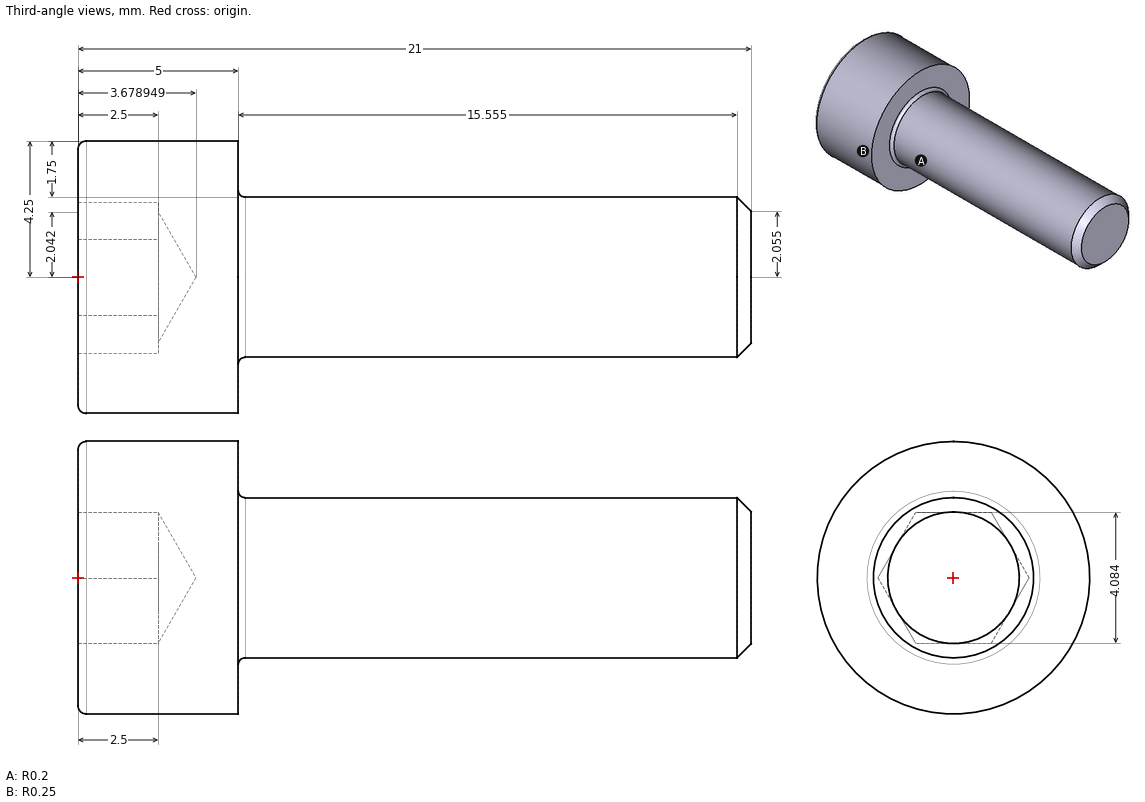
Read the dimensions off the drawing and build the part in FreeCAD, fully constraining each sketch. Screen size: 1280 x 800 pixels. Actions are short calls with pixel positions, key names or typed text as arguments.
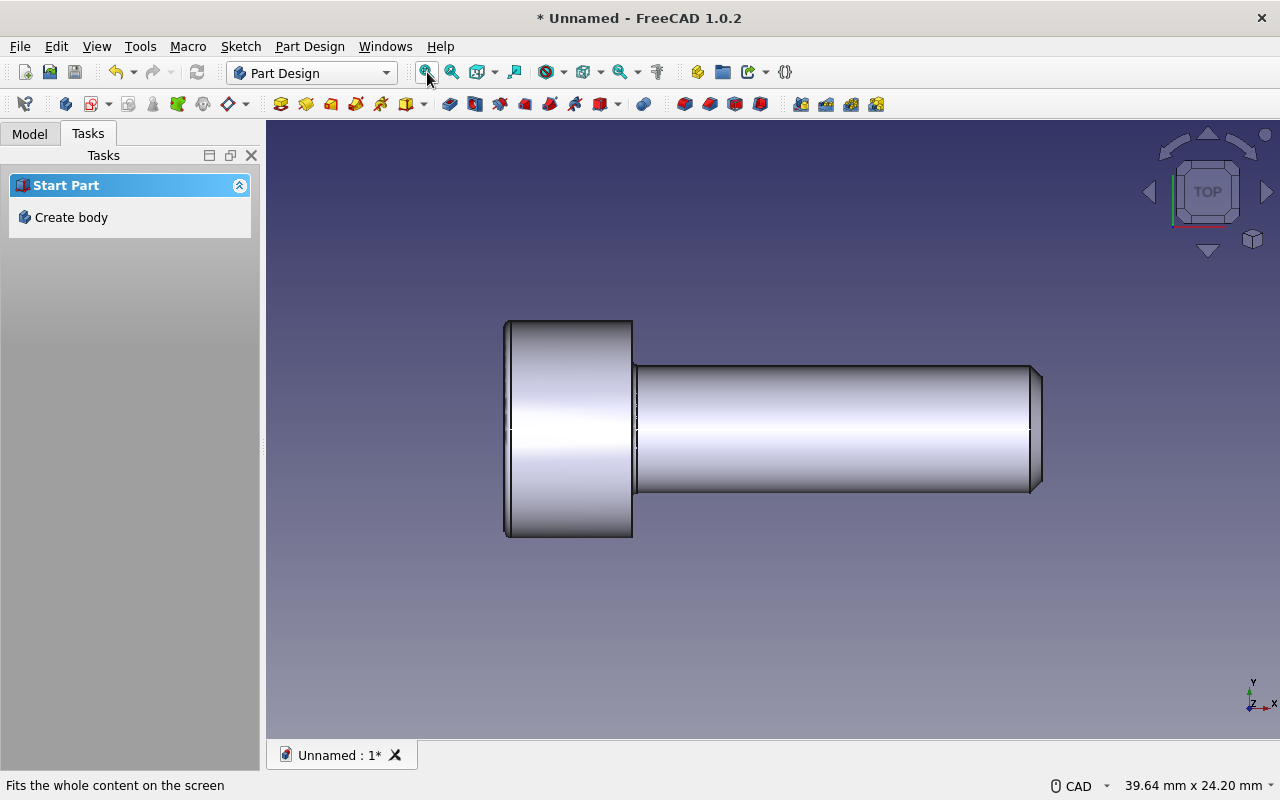
key(6)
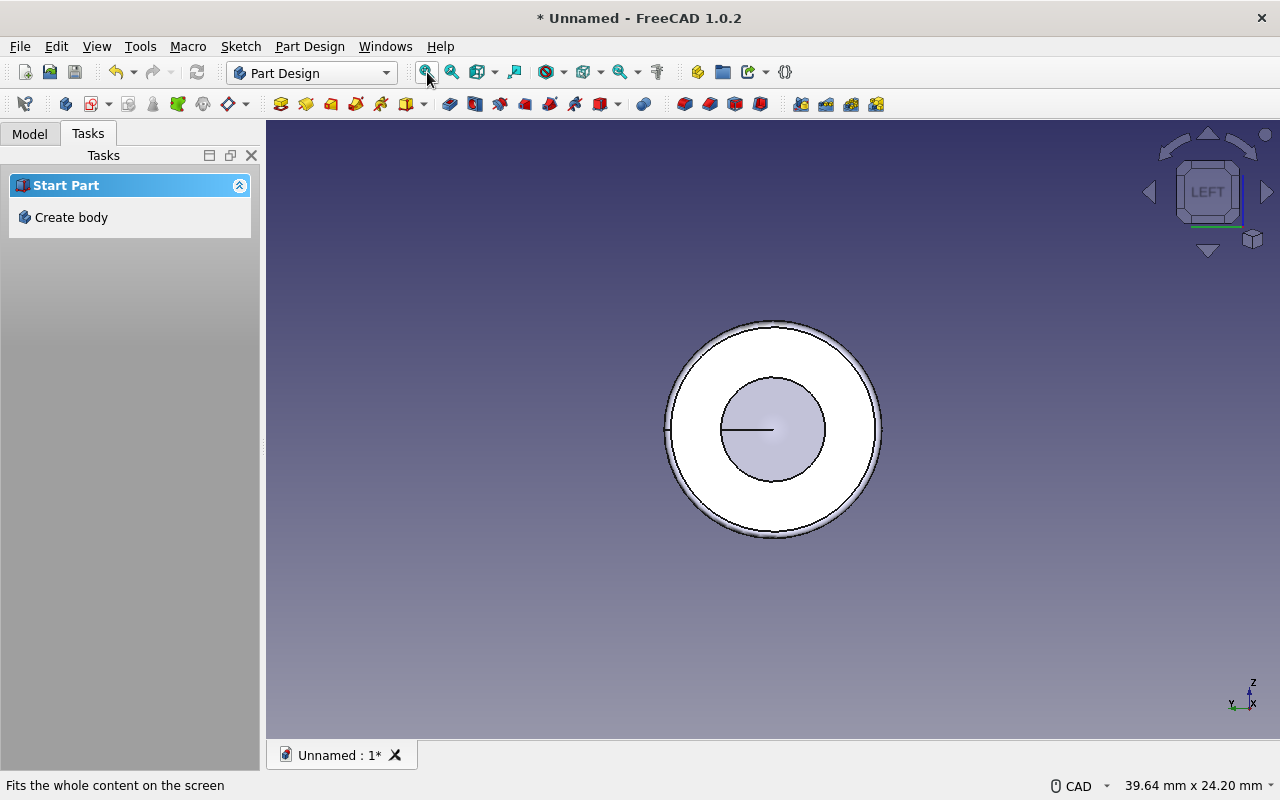
click(427, 72)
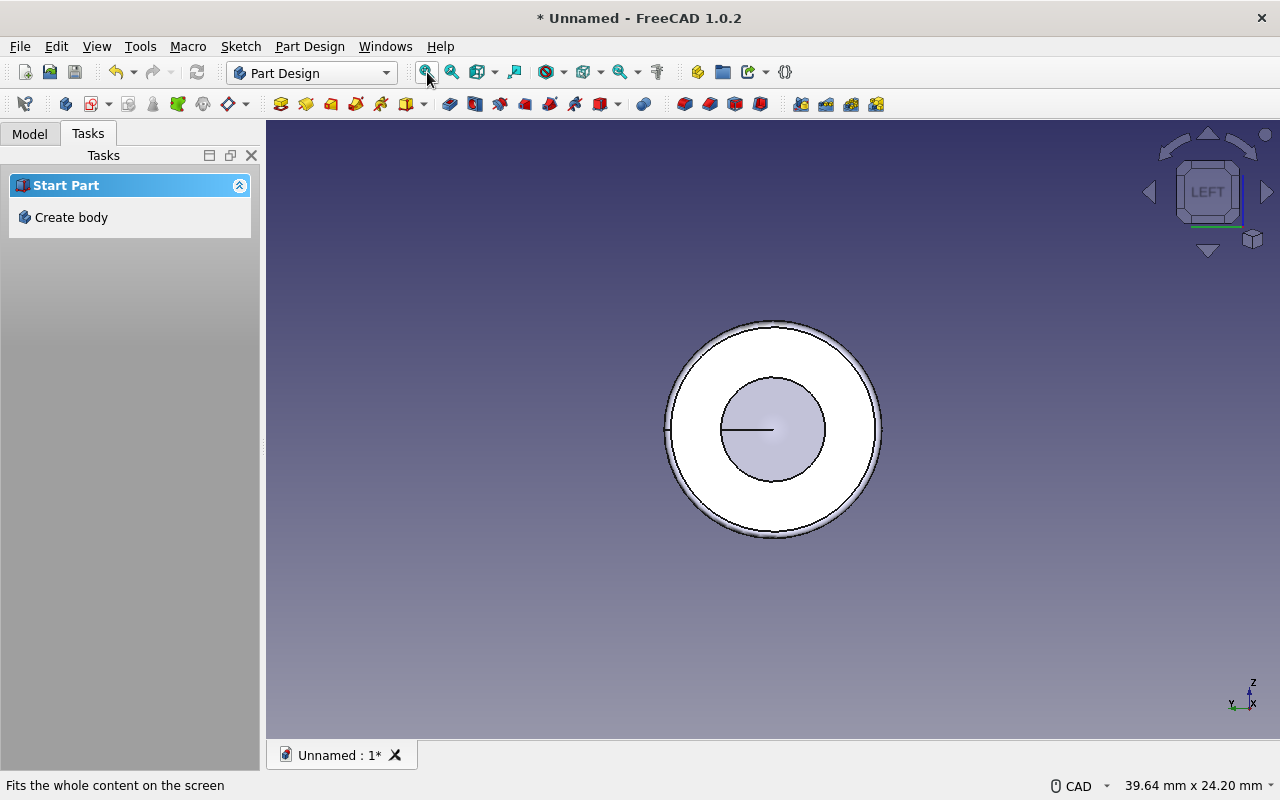
click(831, 487)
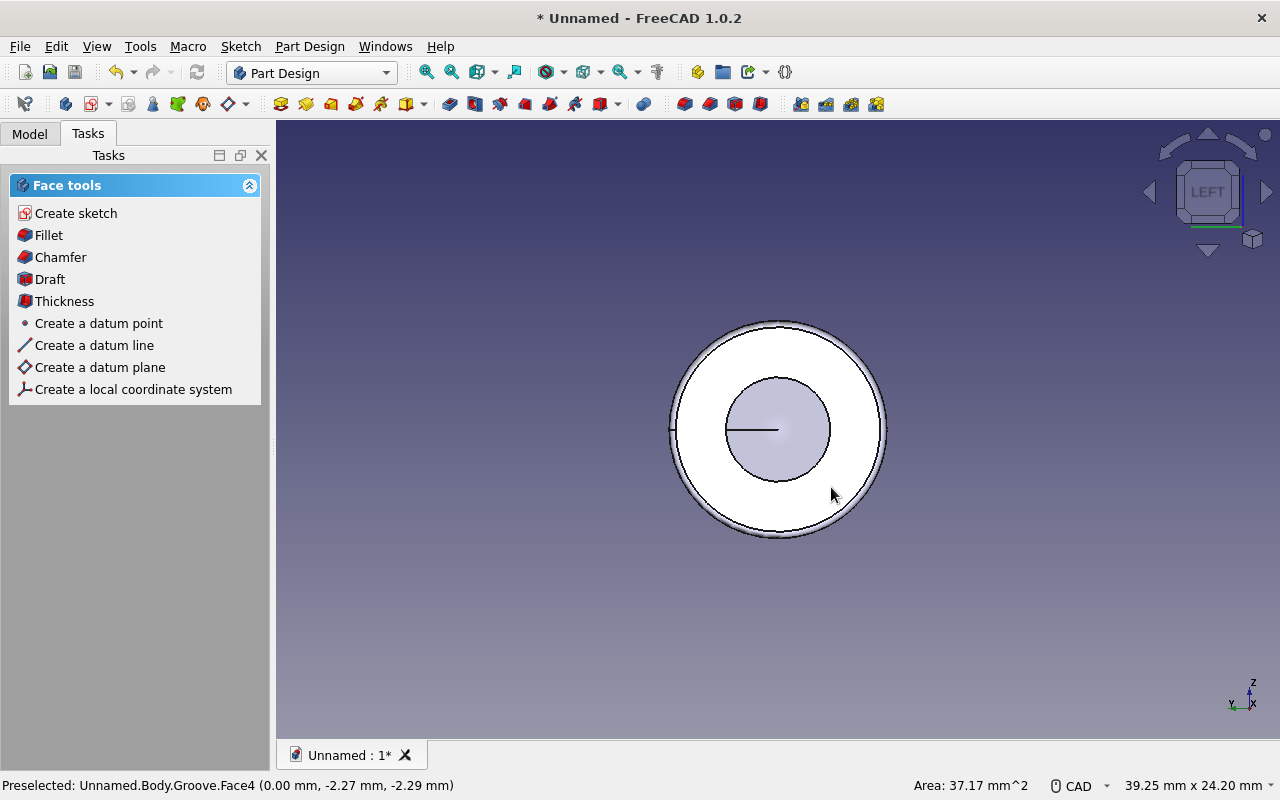
click(90, 104)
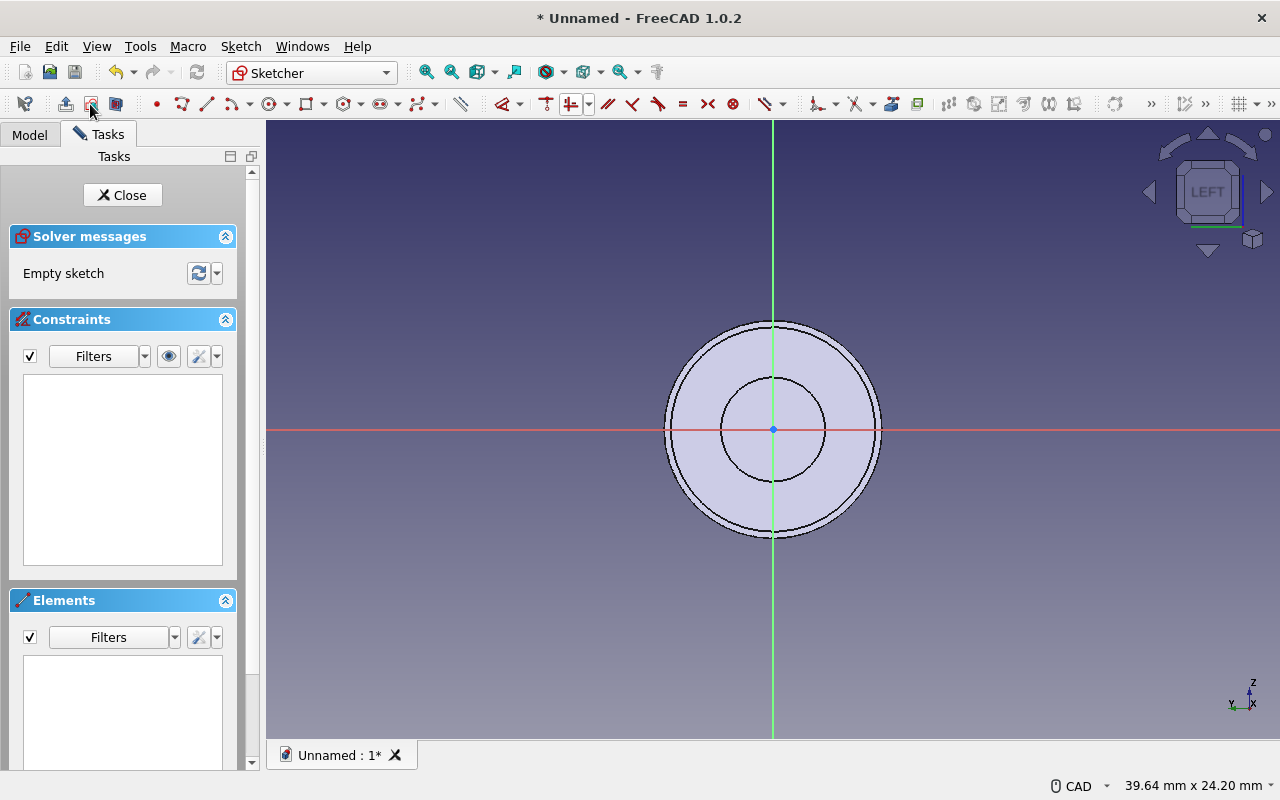
scroll(795, 430, up, 7)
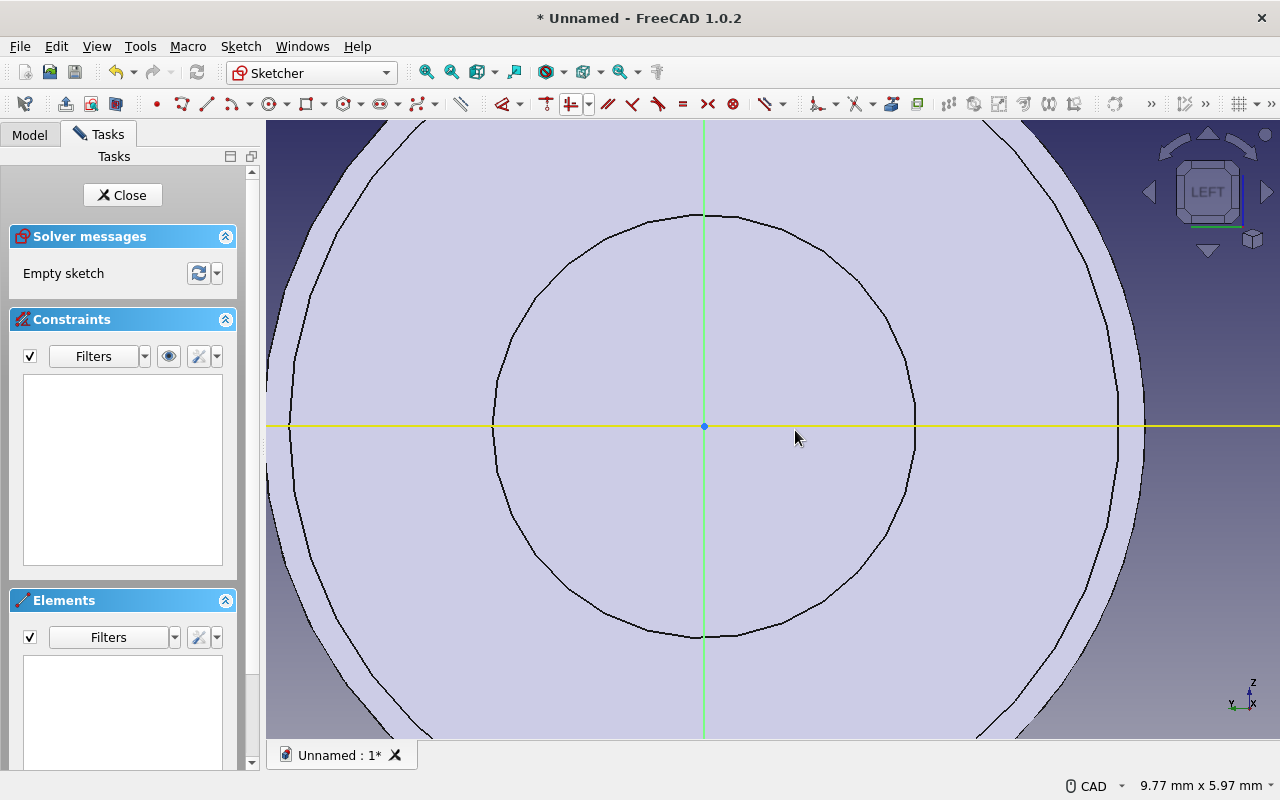
click(342, 104)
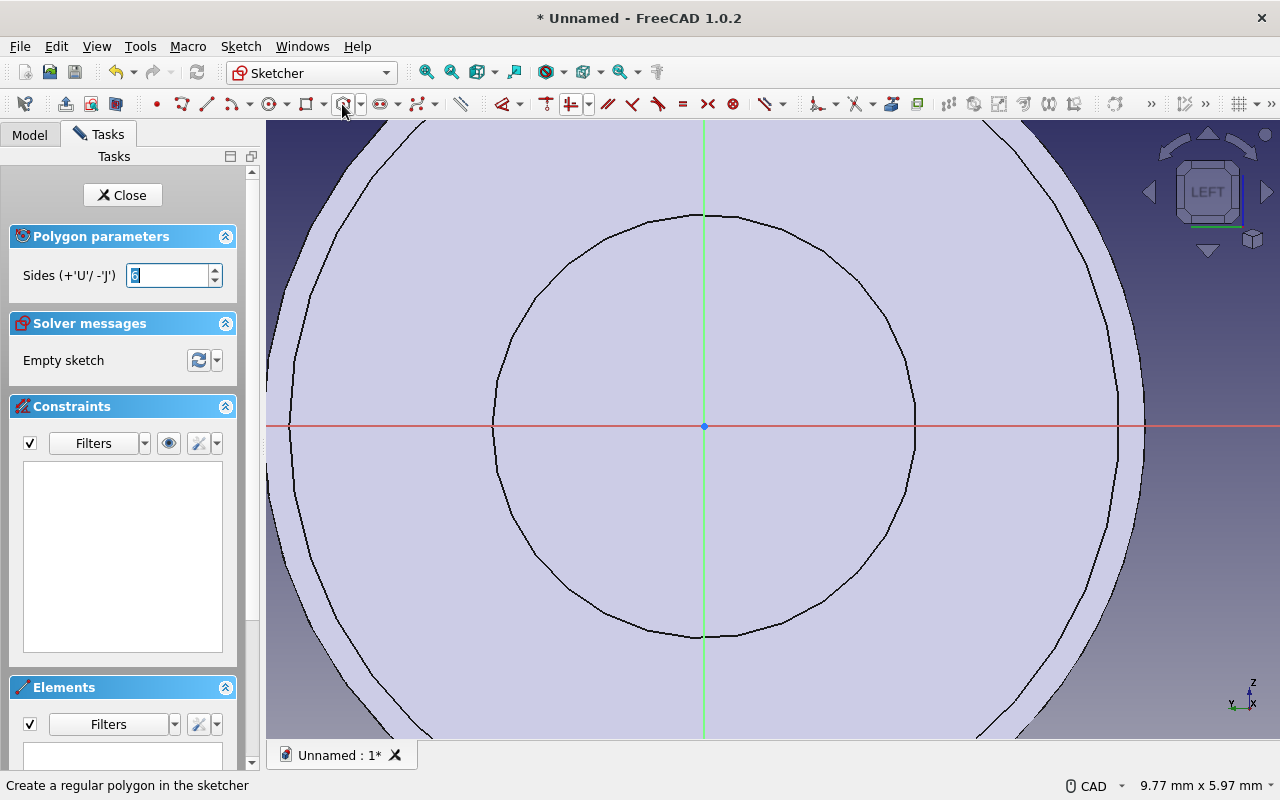
click(704, 426)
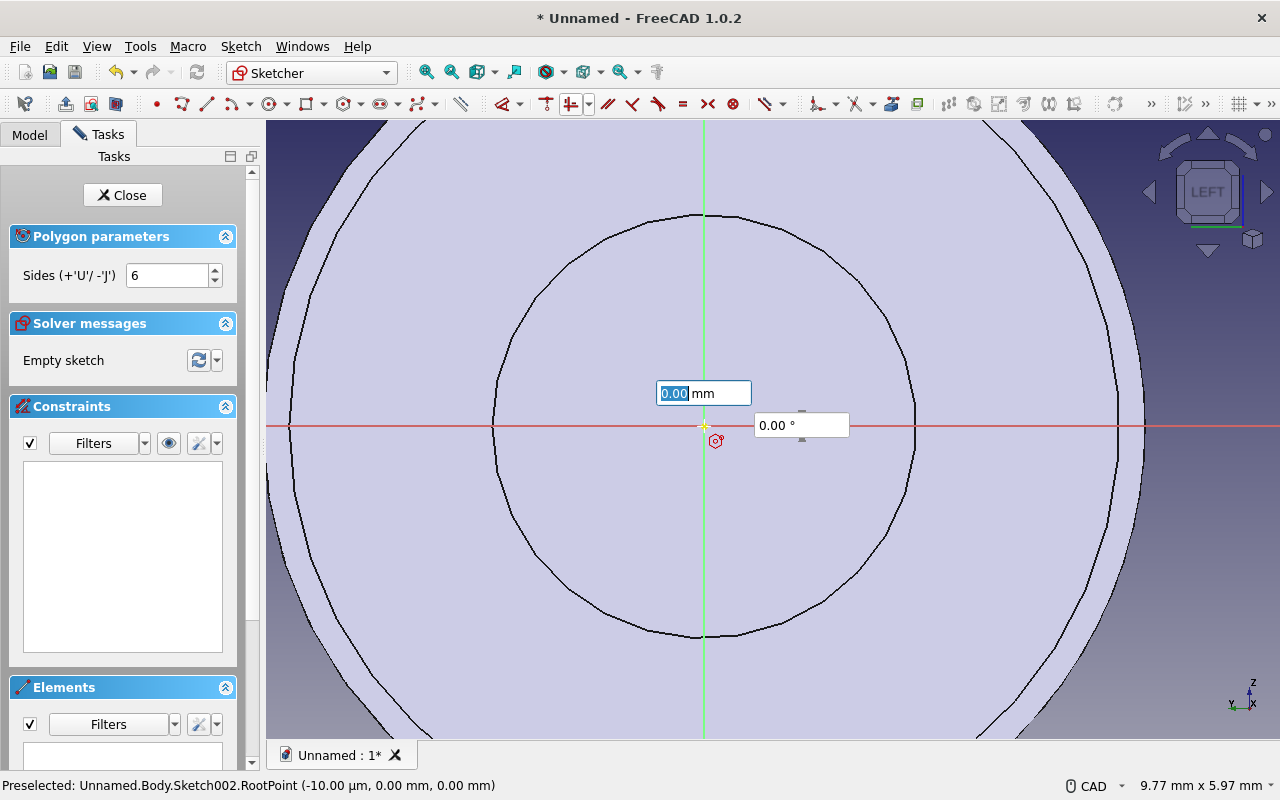
click(460, 426)
right_click(460, 426)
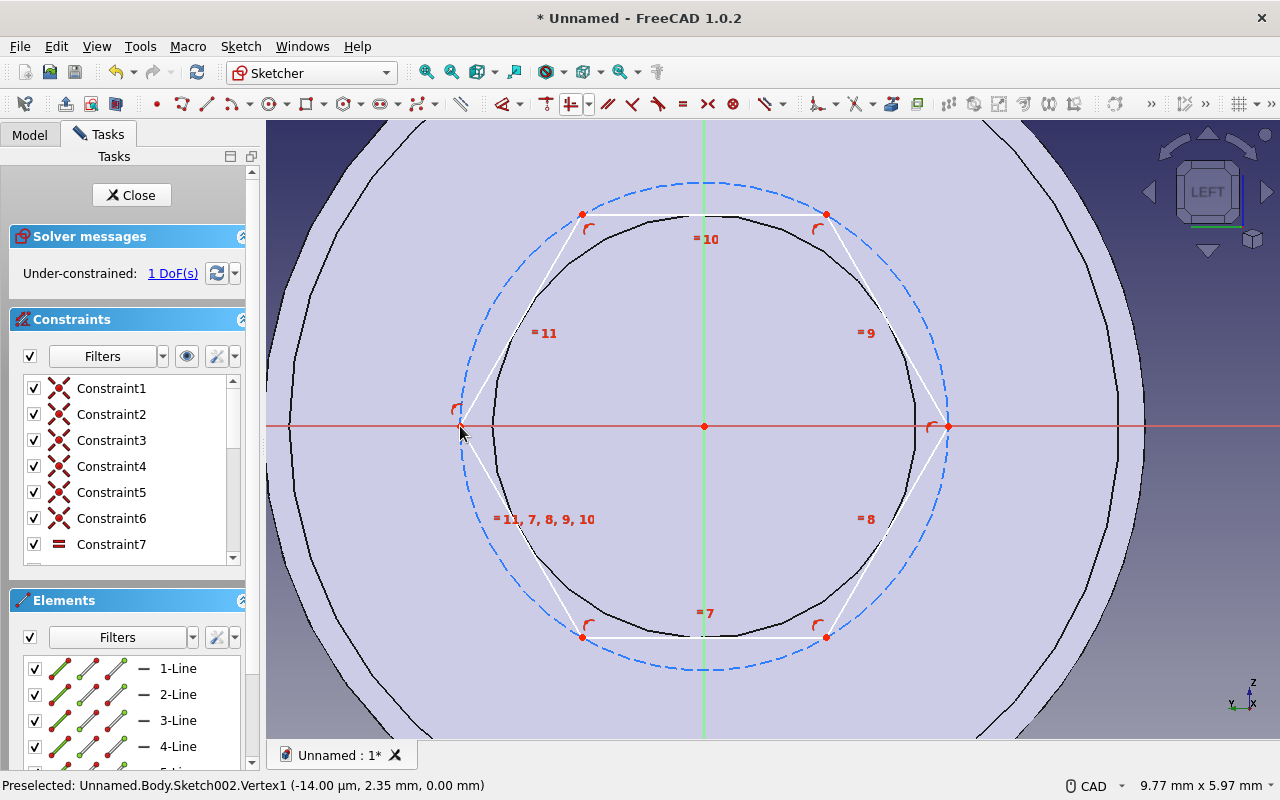
click(502, 104)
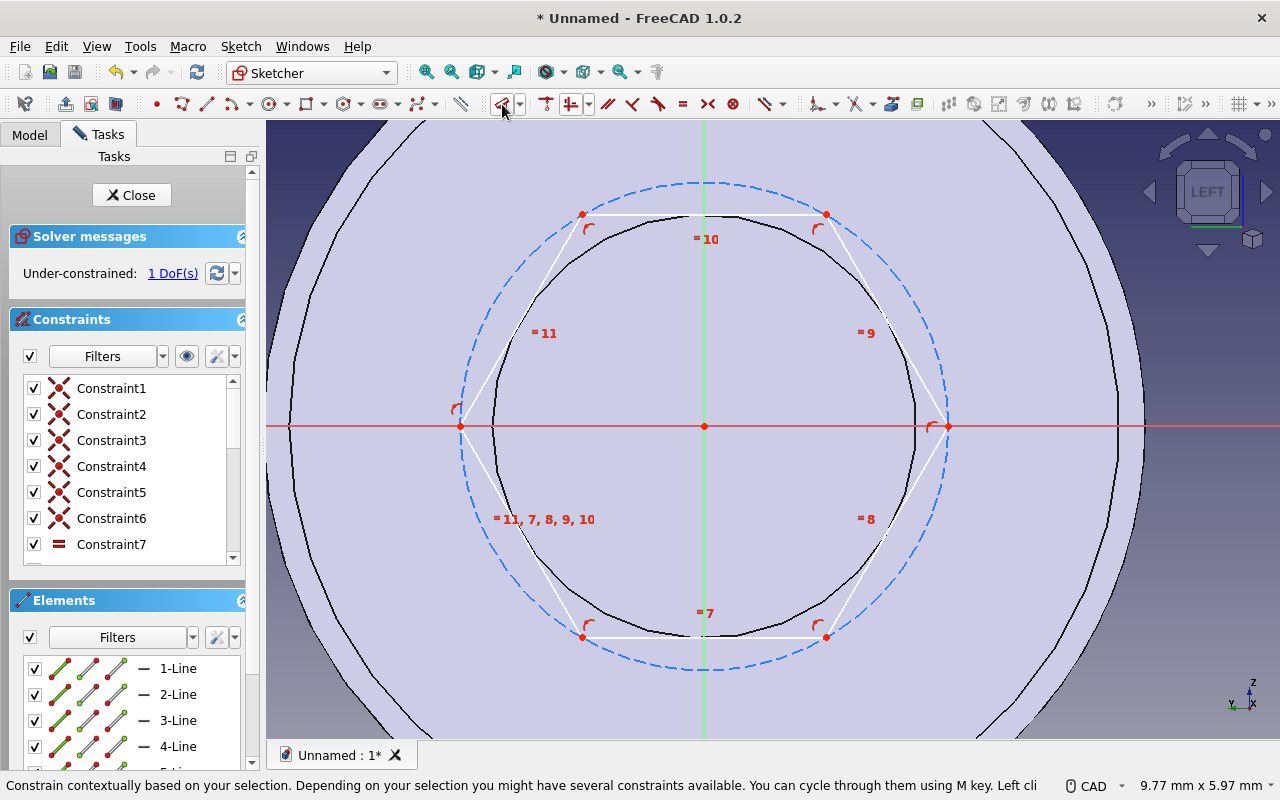
click(582, 638)